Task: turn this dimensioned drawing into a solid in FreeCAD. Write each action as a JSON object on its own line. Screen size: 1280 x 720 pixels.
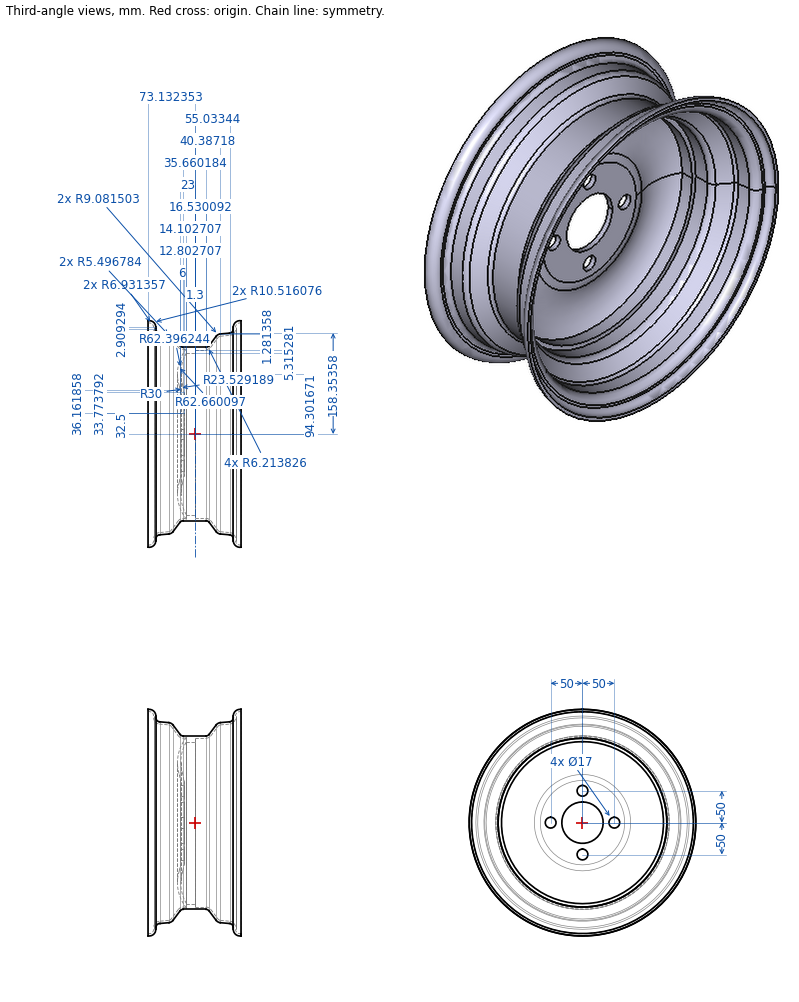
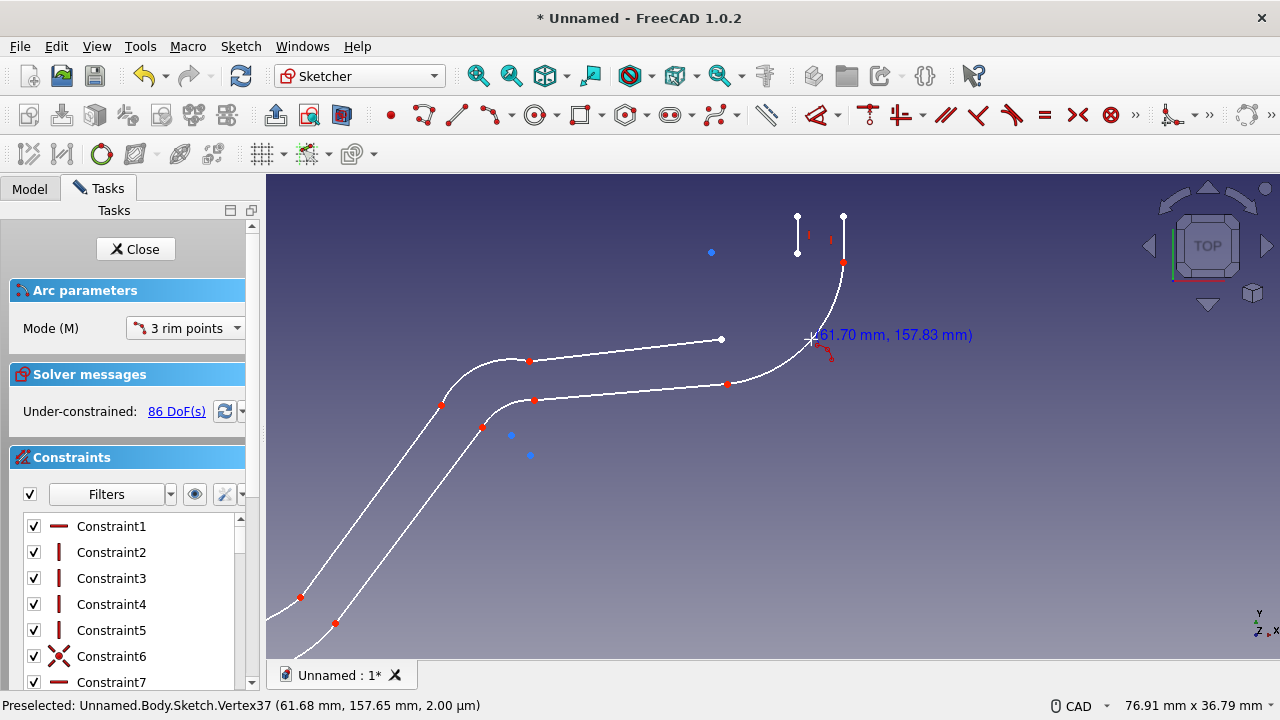
{"action": "left_click", "coordinate": [844, 216]}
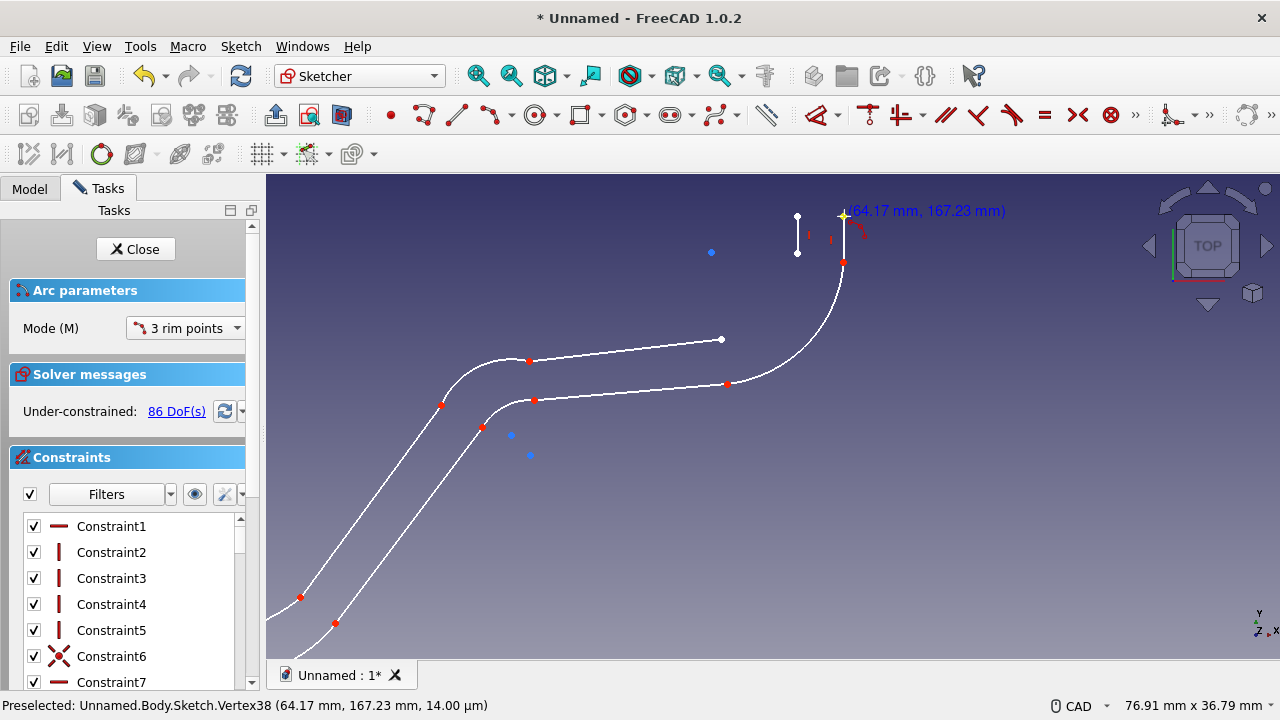
{"action": "scroll", "coordinate": [815, 286], "scroll_direction": "down", "scroll_amount": 10}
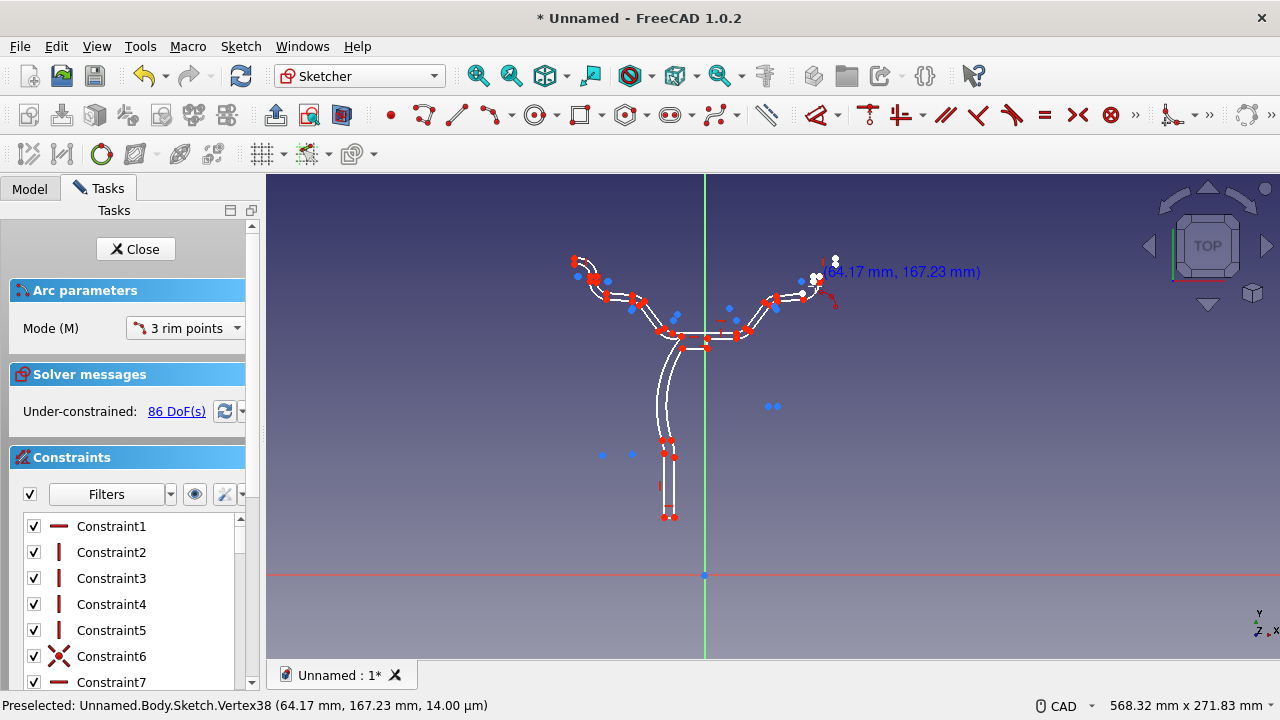
{"action": "scroll", "coordinate": [835, 264], "scroll_direction": "up", "scroll_amount": 8}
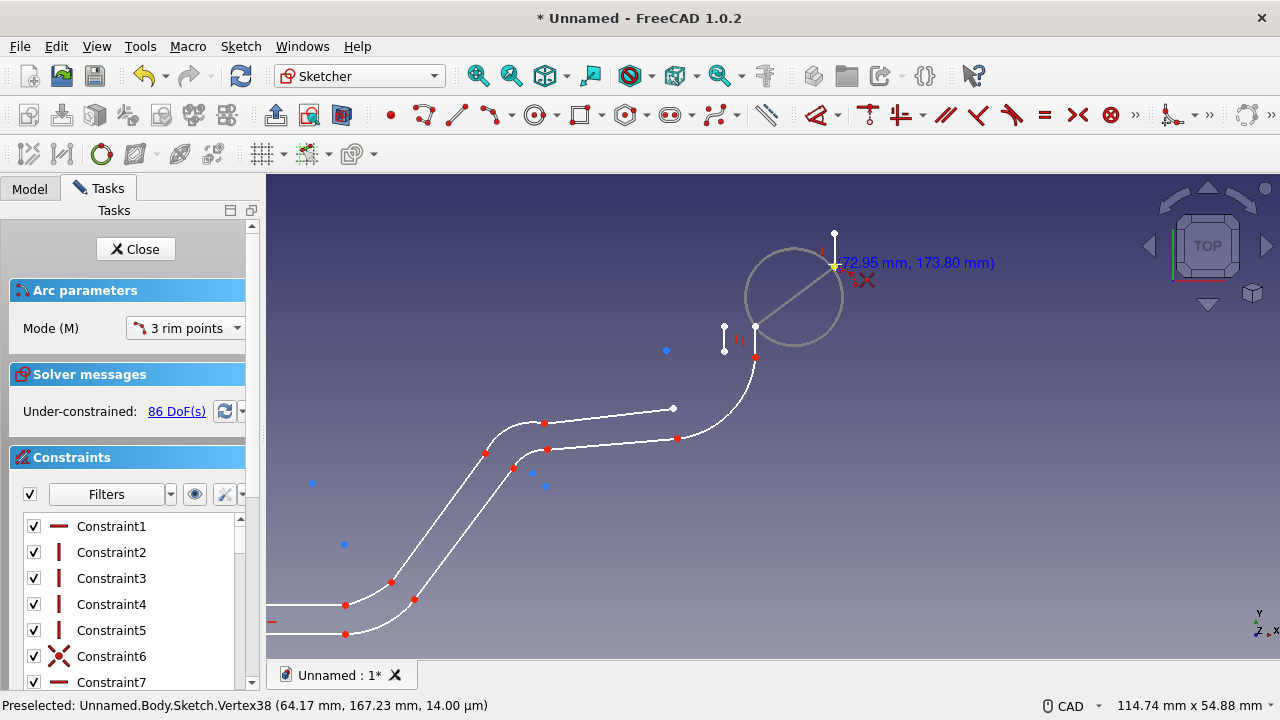
{"action": "left_click", "coordinate": [835, 267]}
{"action": "left_click", "coordinate": [781, 275]}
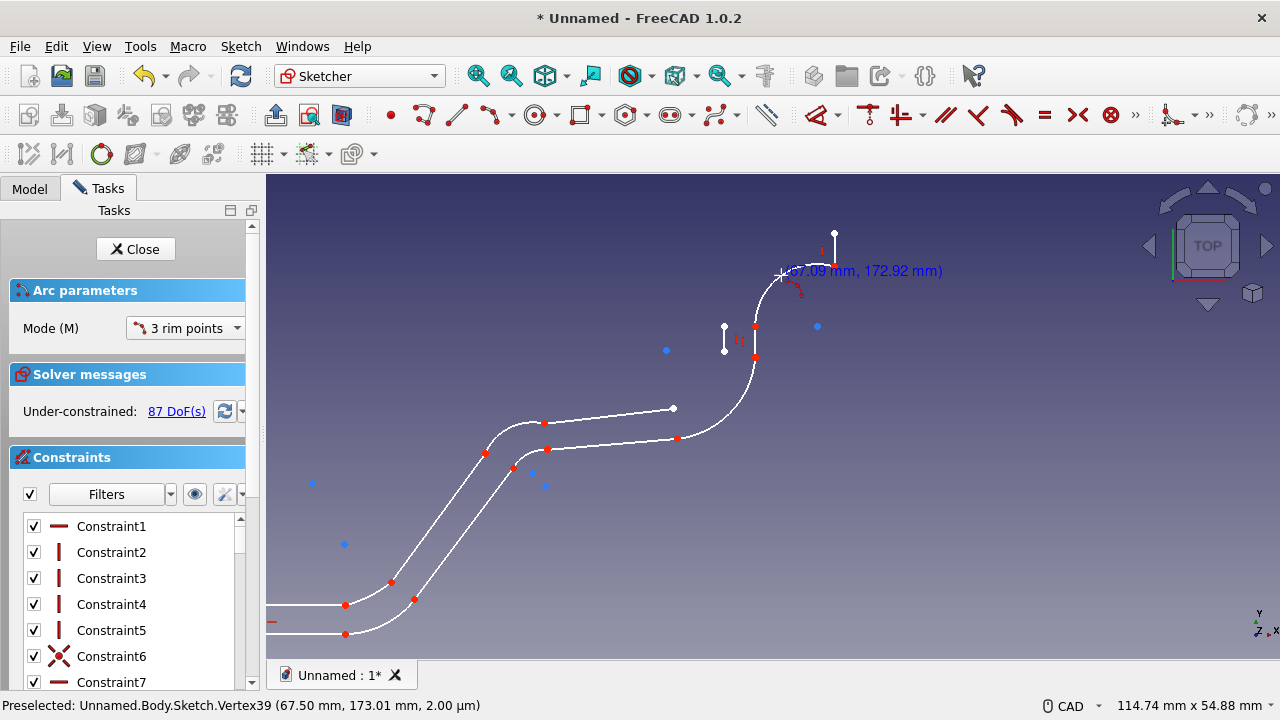
{"action": "left_click", "coordinate": [835, 234]}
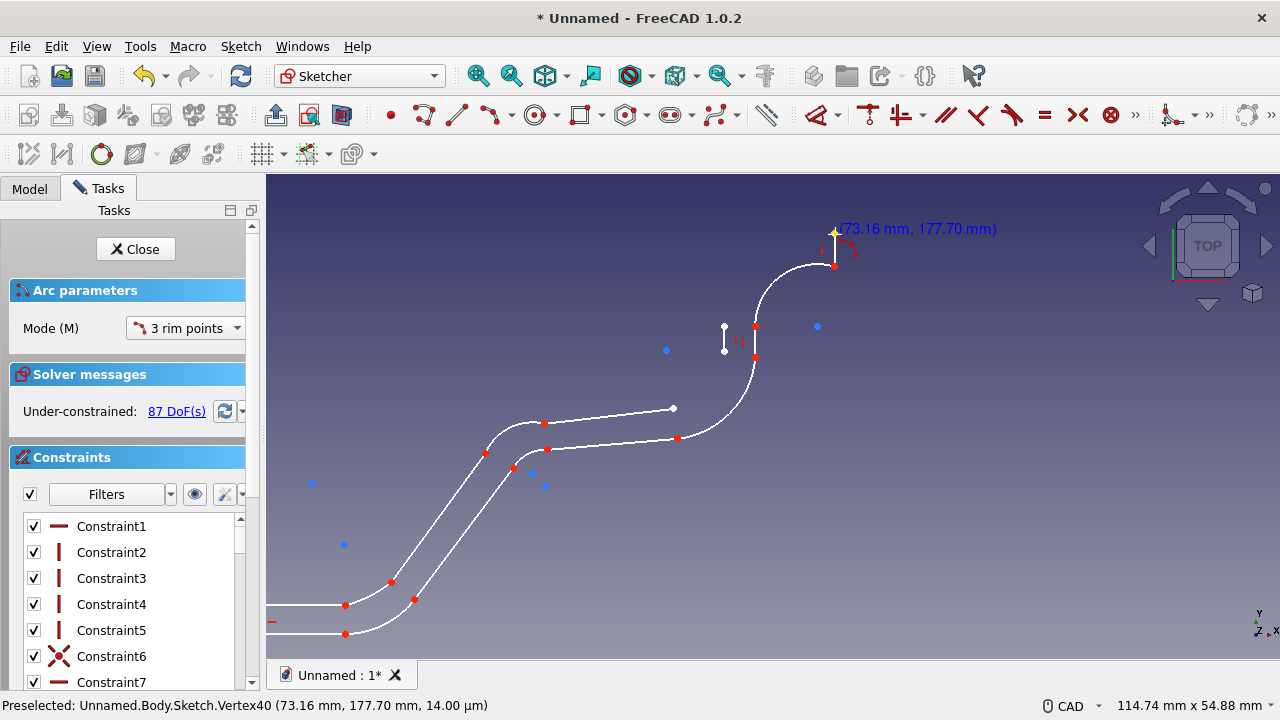
{"action": "scroll", "coordinate": [725, 324], "scroll_direction": "up", "scroll_amount": 2}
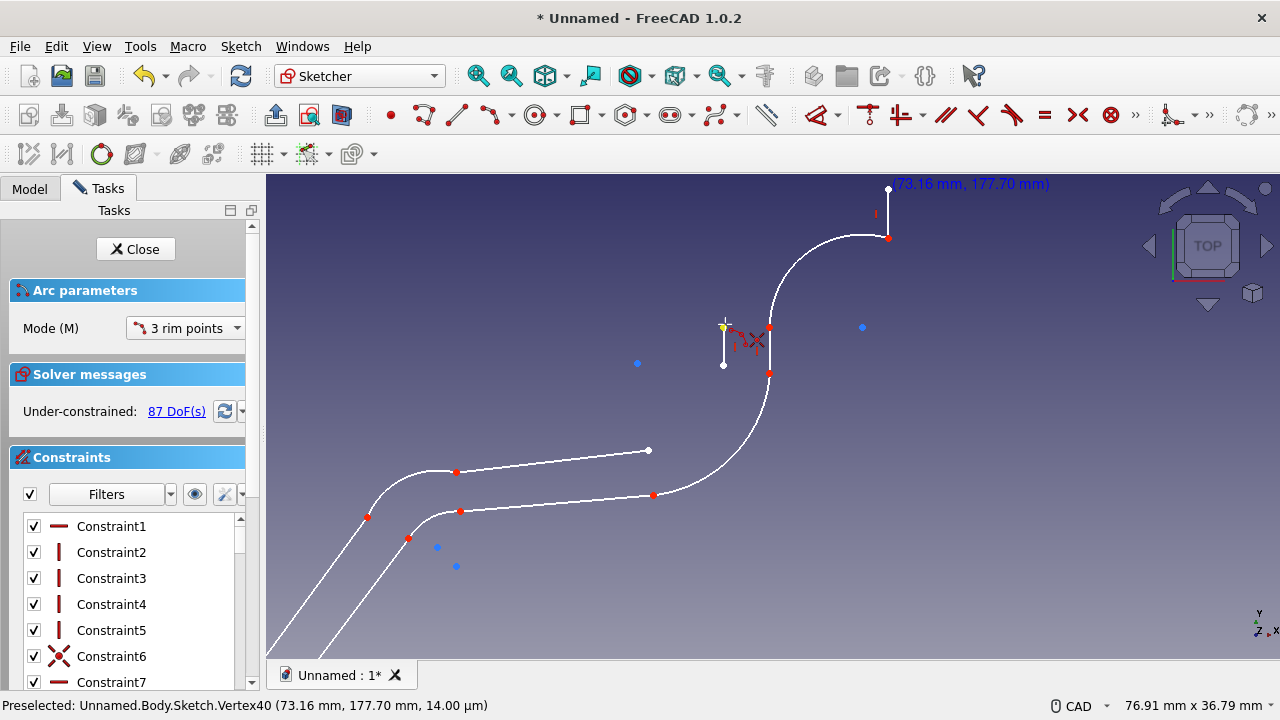
{"action": "left_click", "coordinate": [724, 327]}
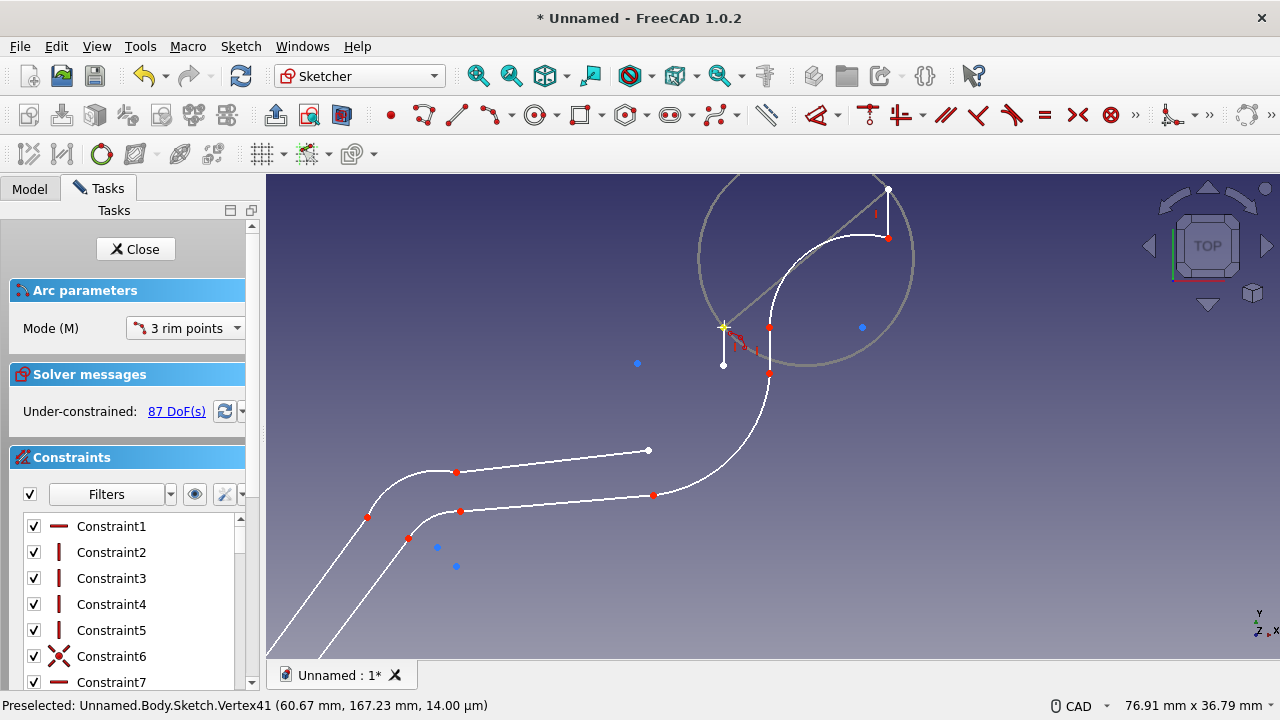
{"action": "scroll", "coordinate": [827, 269], "scroll_direction": "down", "scroll_amount": 10}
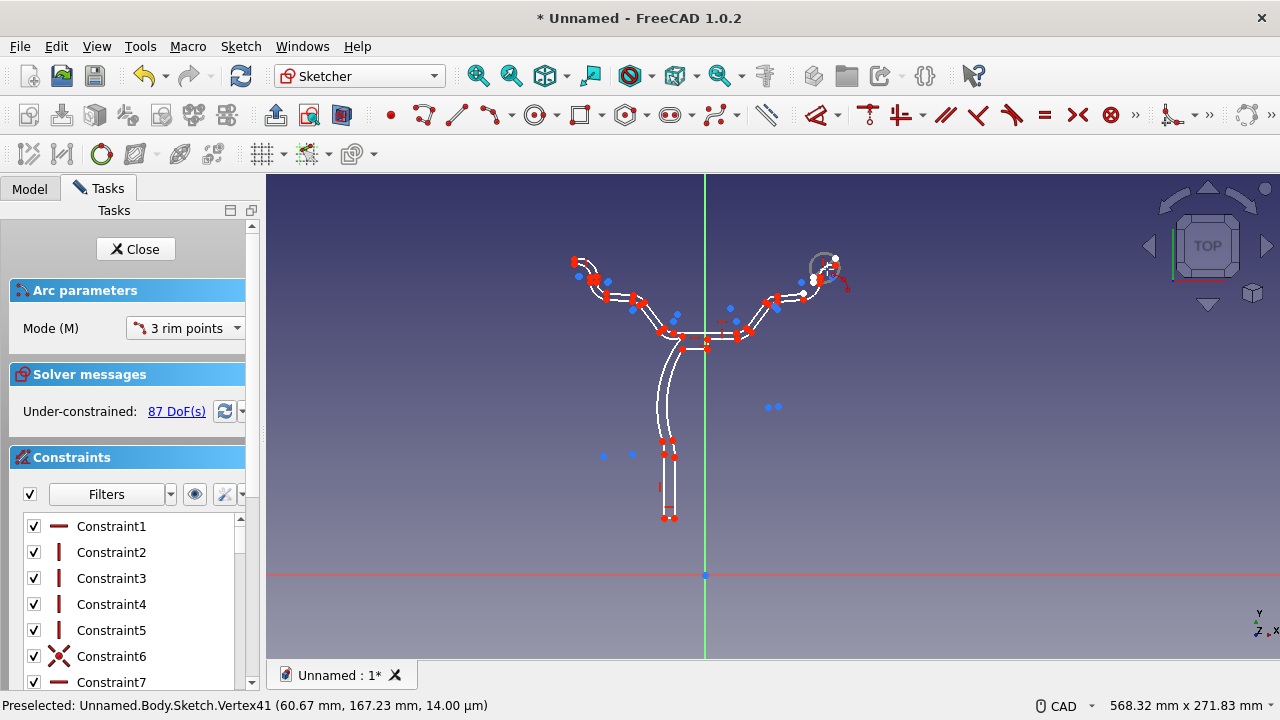
{"action": "scroll", "coordinate": [818, 265], "scroll_direction": "up", "scroll_amount": 5}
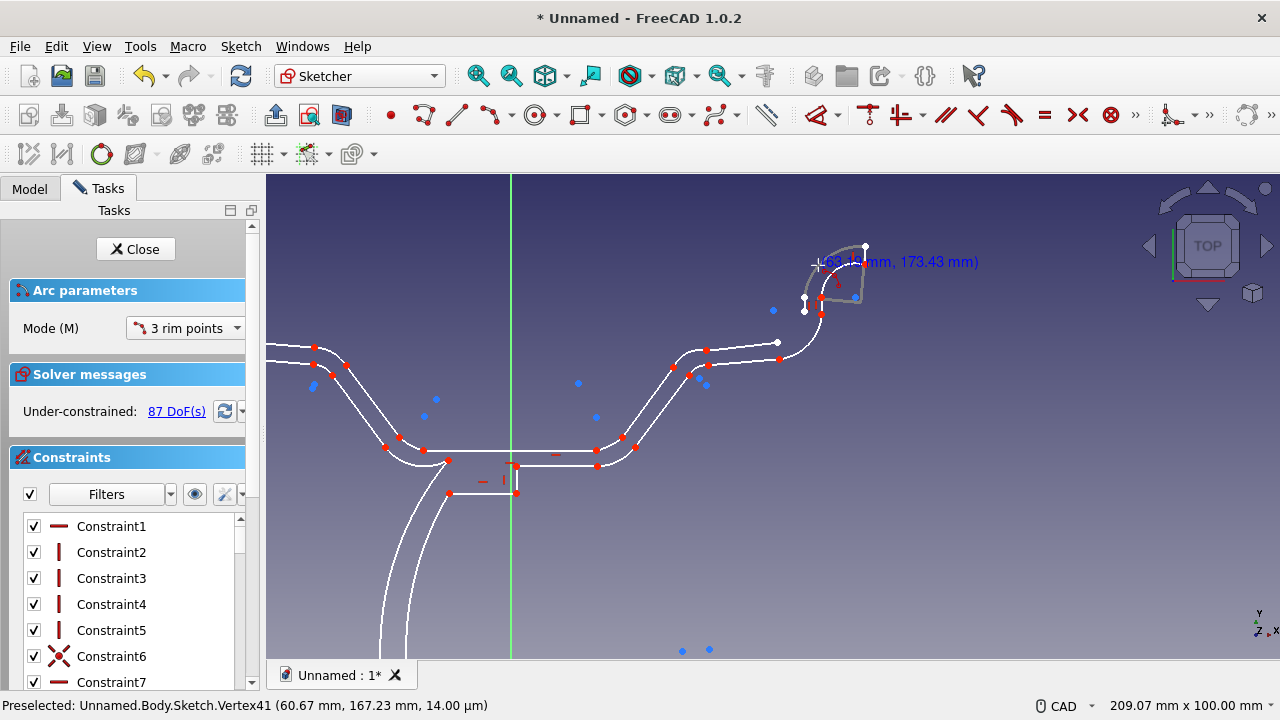
{"action": "left_click", "coordinate": [817, 263]}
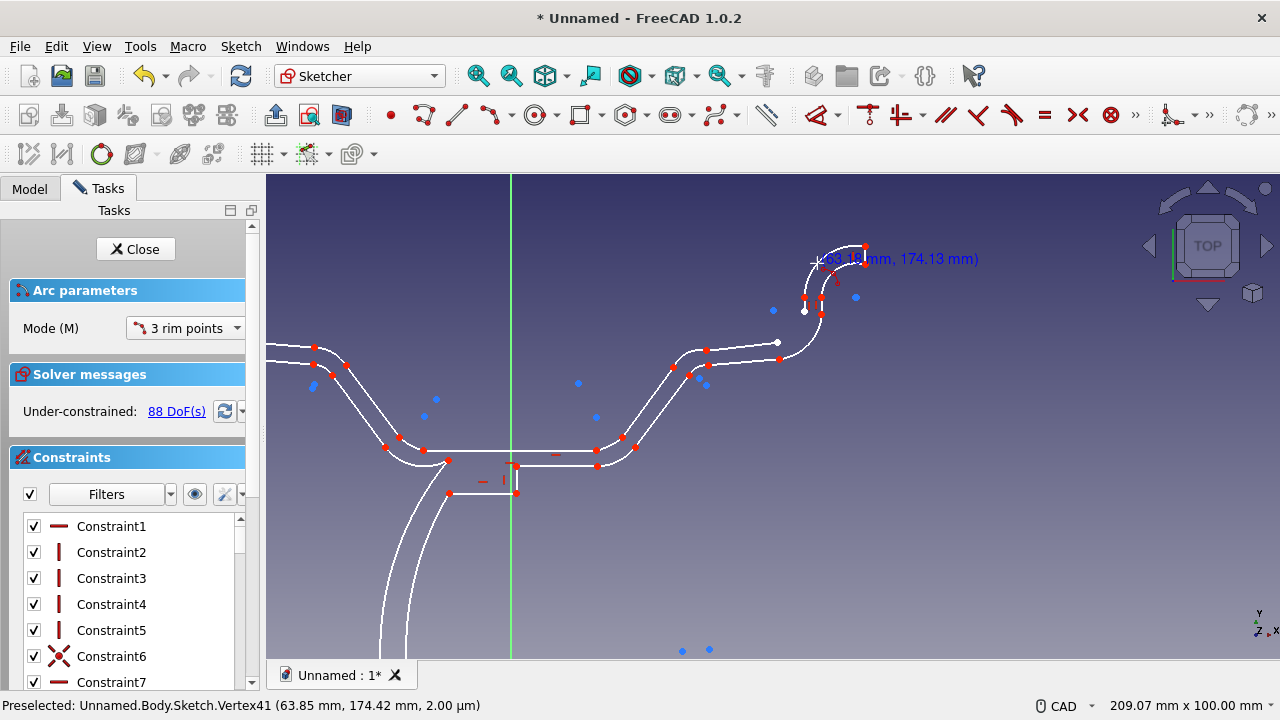
{"action": "scroll", "coordinate": [805, 310], "scroll_direction": "up", "scroll_amount": 5}